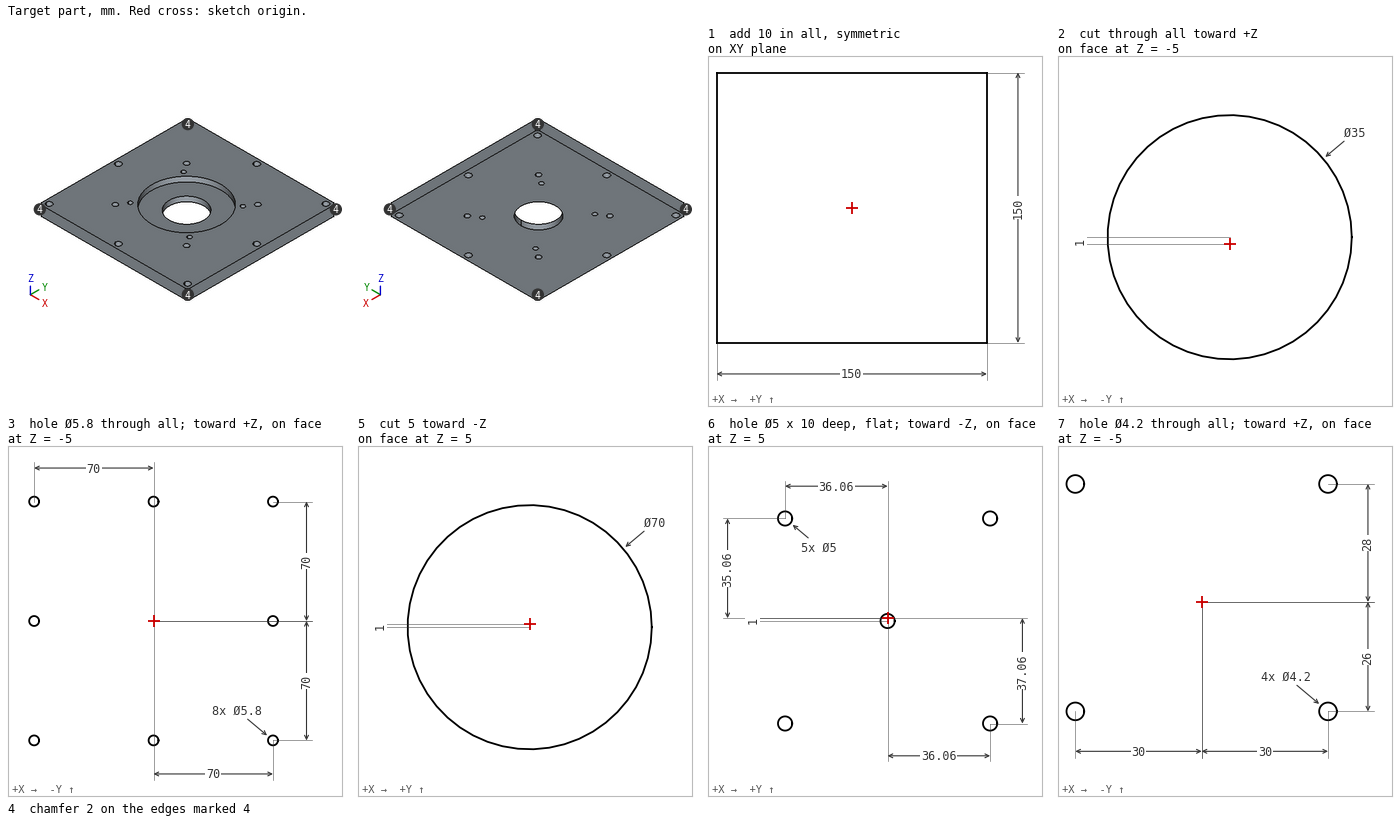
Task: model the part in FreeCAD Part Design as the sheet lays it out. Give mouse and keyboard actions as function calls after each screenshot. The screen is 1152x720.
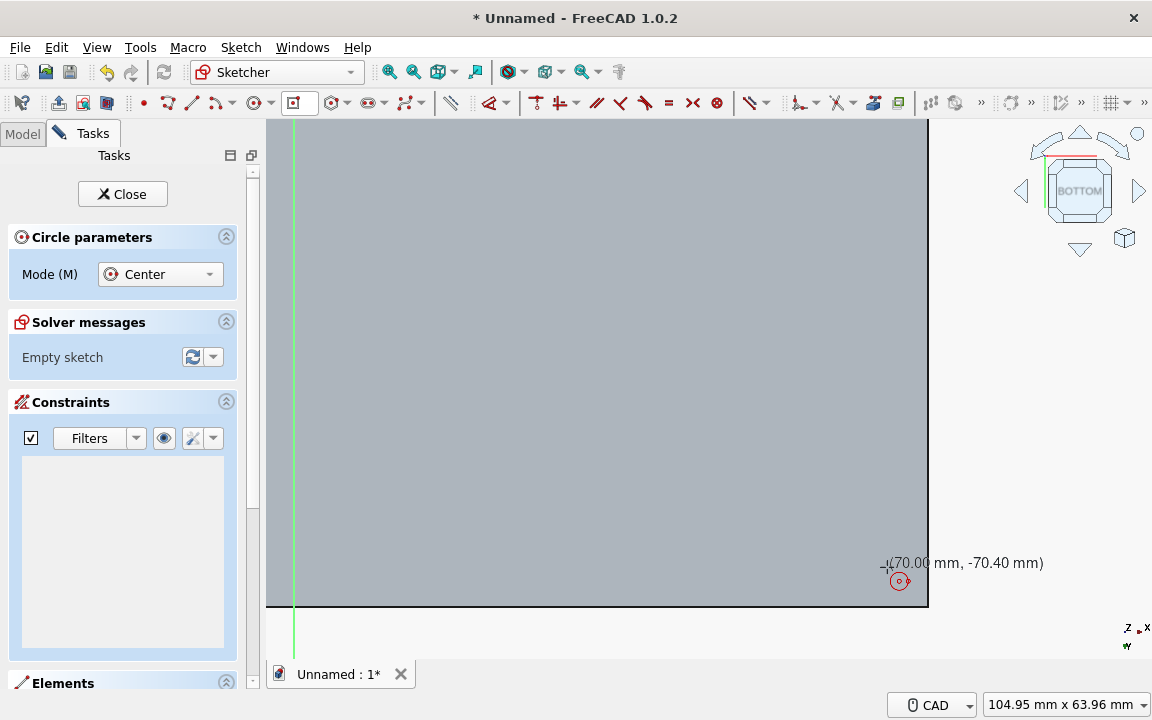
click(885, 565)
move(903, 548)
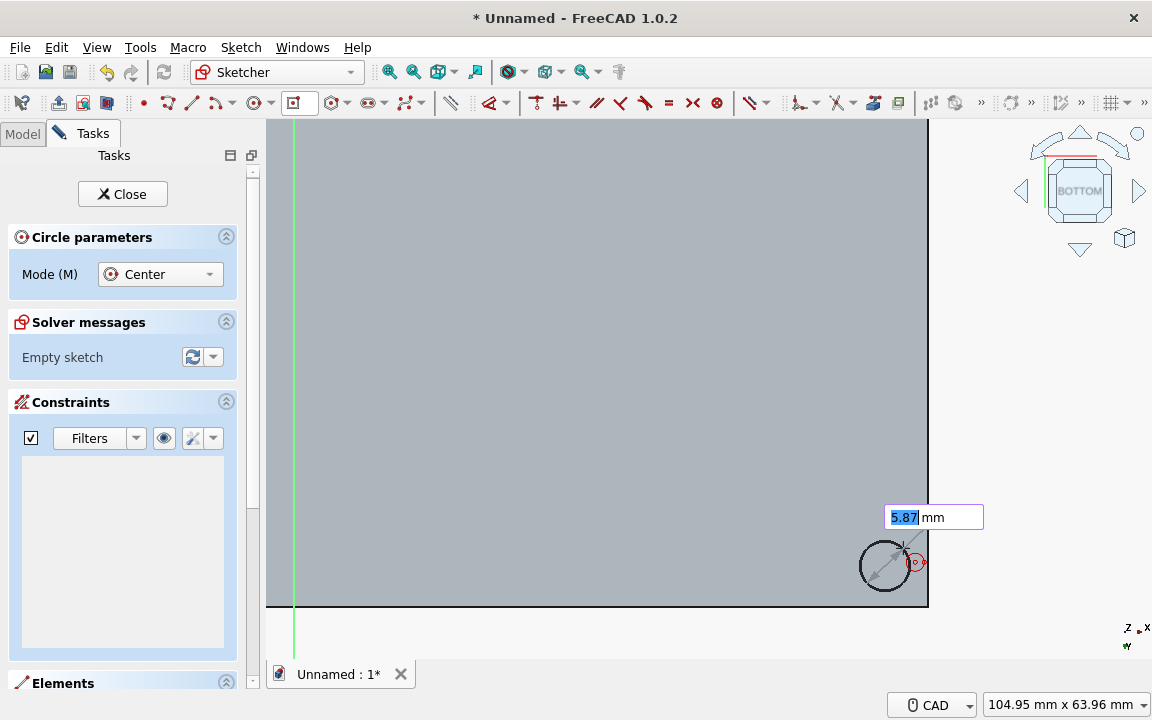
text(5.8)
key(Return)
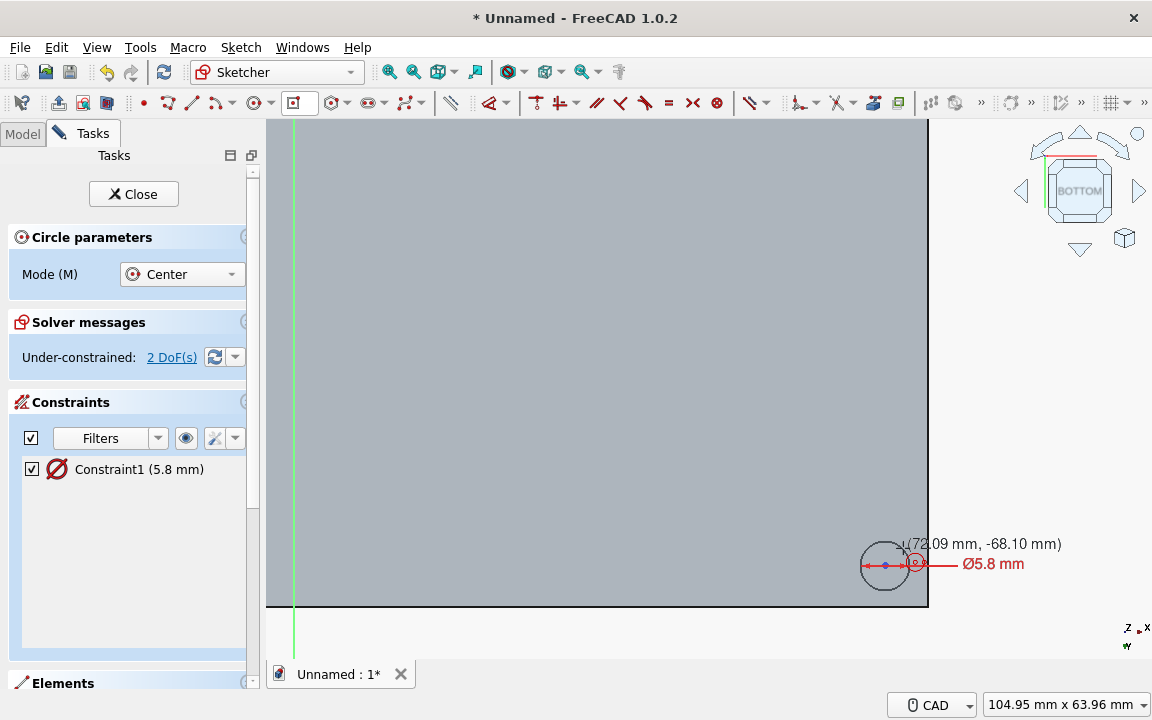
scroll(790, 568, down, 6)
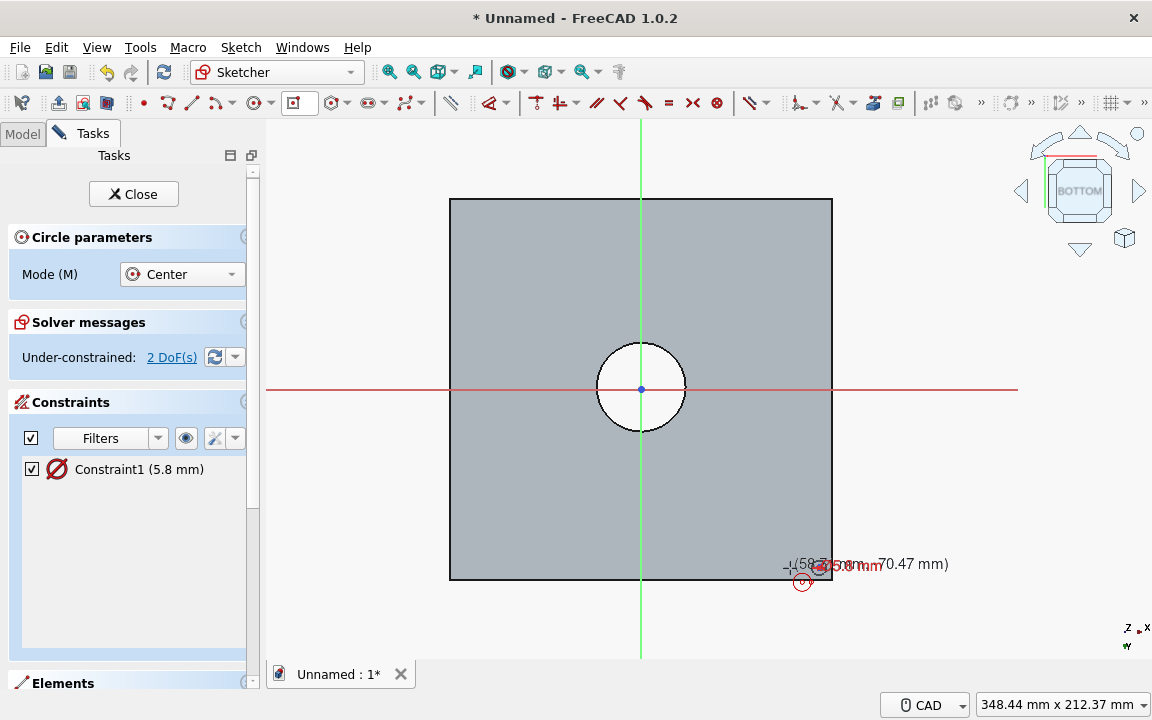
scroll(819, 390, up, 6)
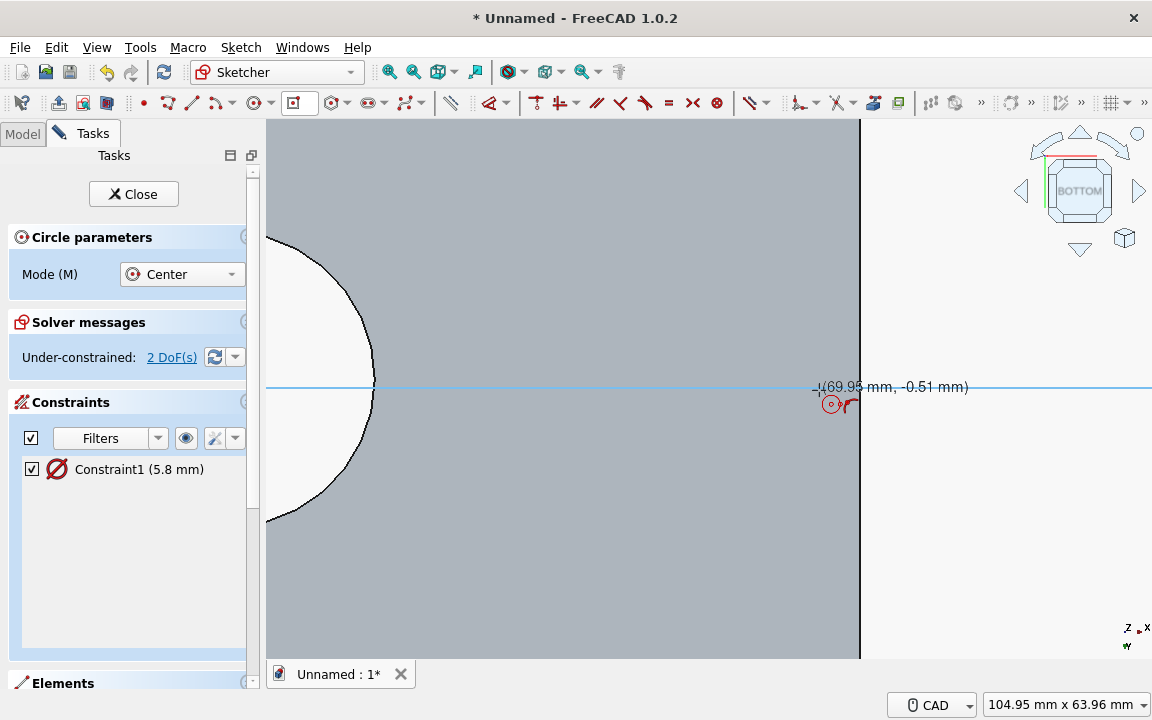
click(818, 388)
move(835, 371)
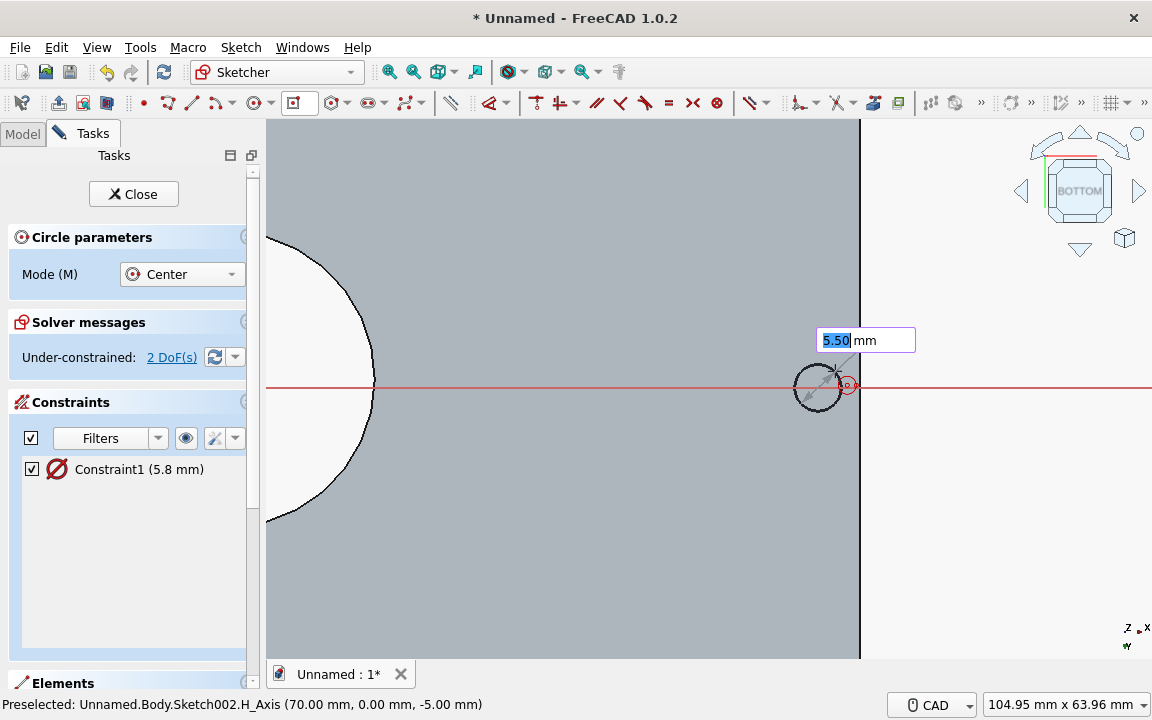
text(5.8)
key(Return)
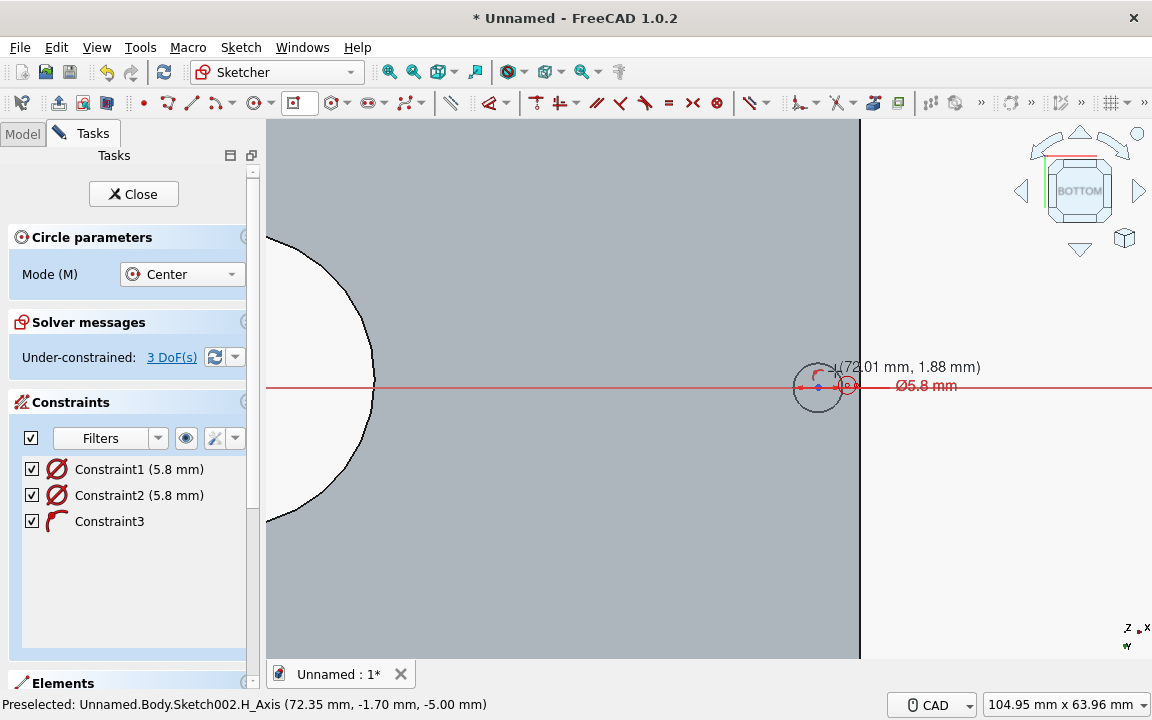
scroll(819, 390, down, 6)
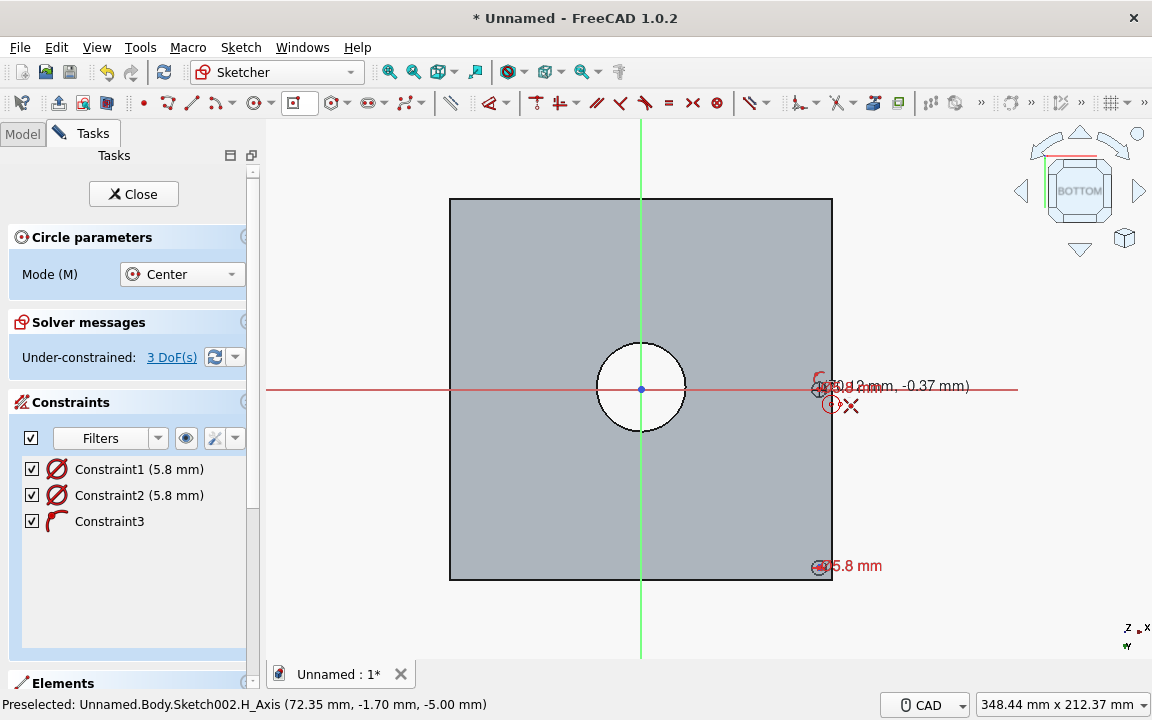
scroll(819, 212, up, 6)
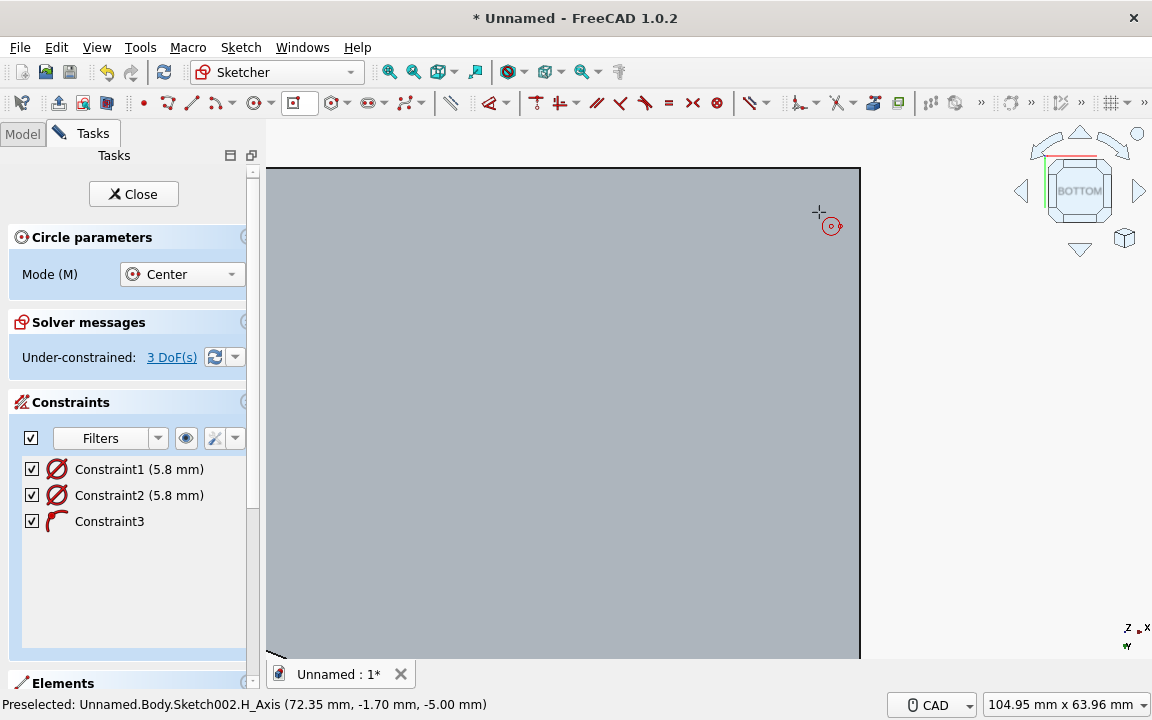
click(818, 211)
move(835, 193)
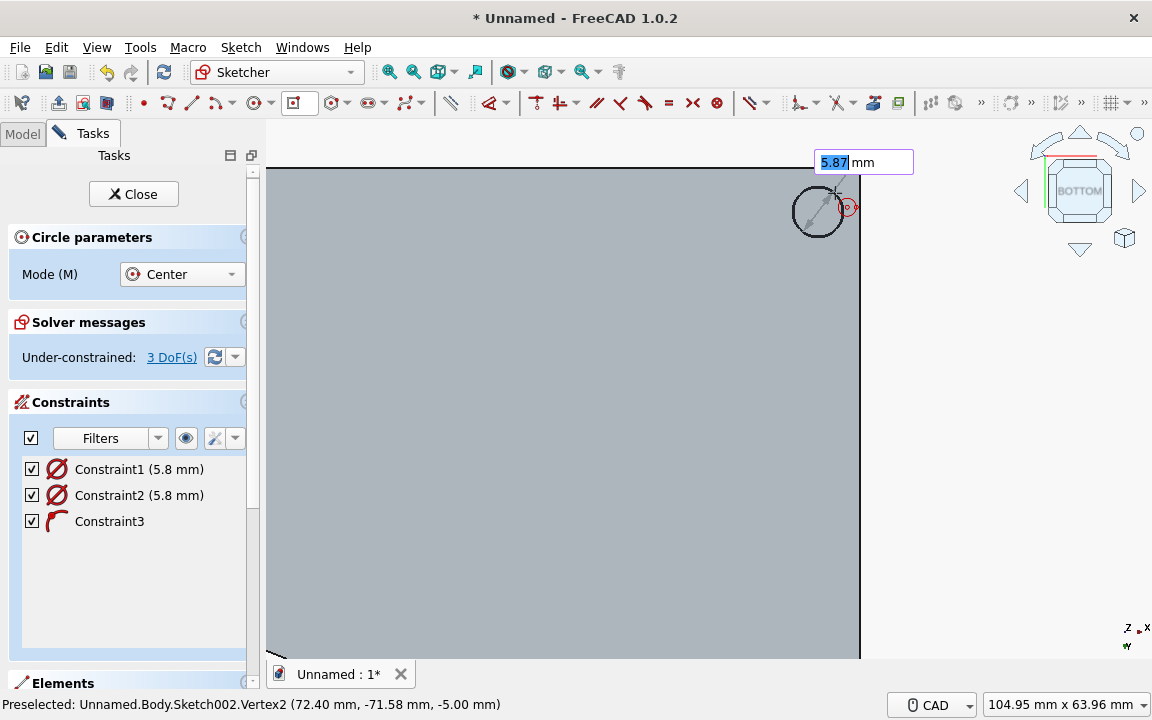
text(5.8)
key(Return)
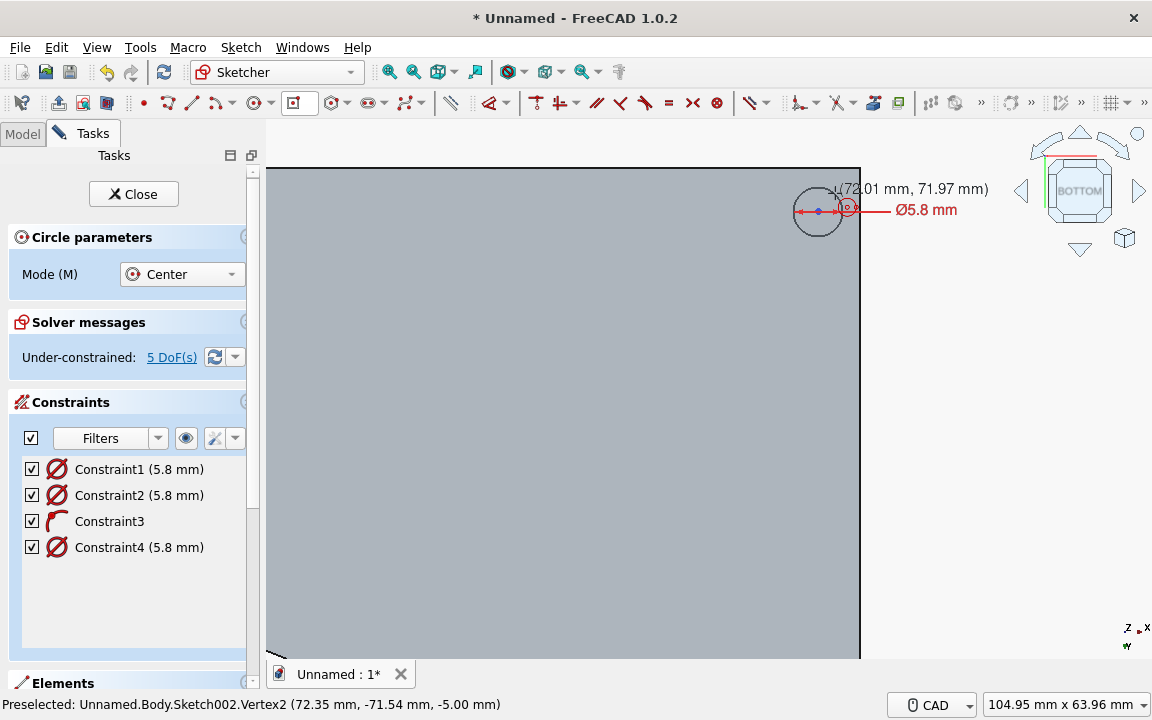
scroll(819, 211, down, 6)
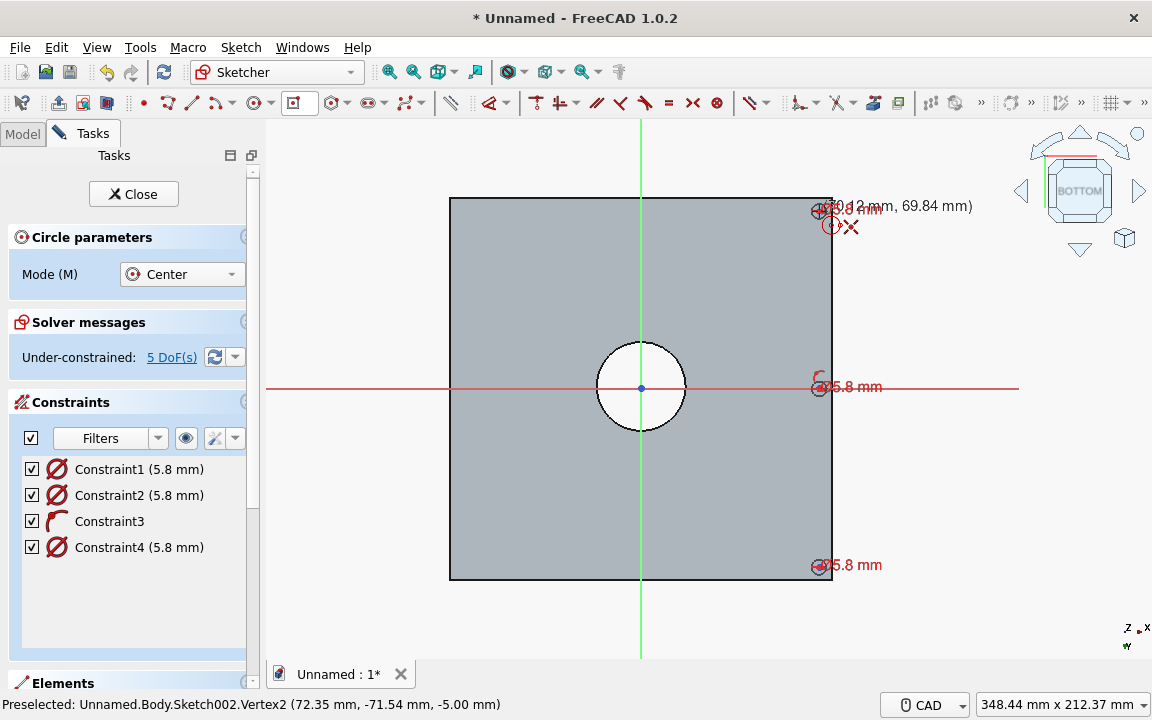
scroll(641, 211, up, 6)